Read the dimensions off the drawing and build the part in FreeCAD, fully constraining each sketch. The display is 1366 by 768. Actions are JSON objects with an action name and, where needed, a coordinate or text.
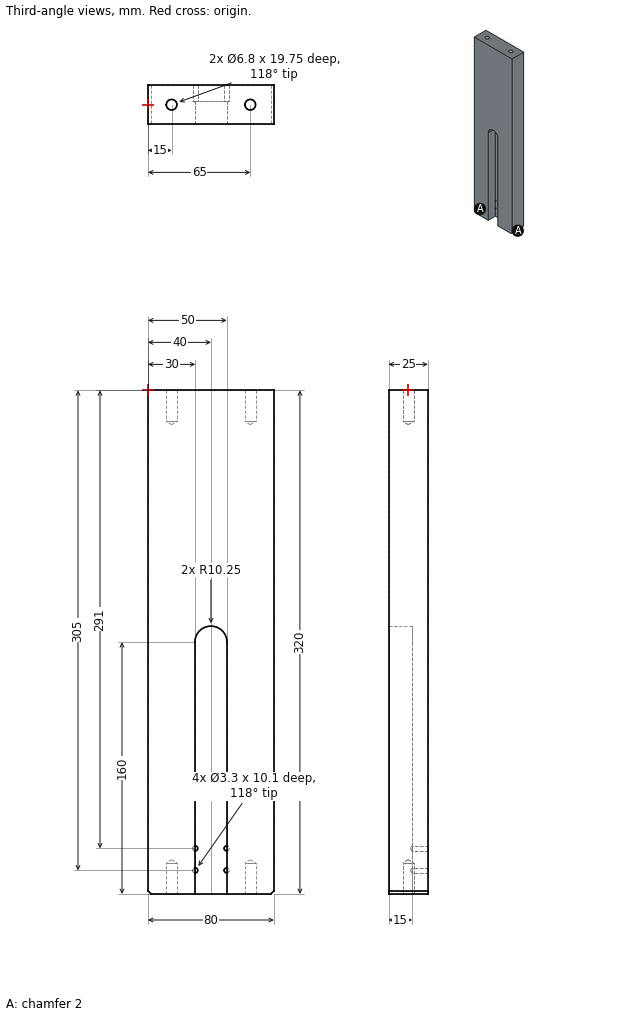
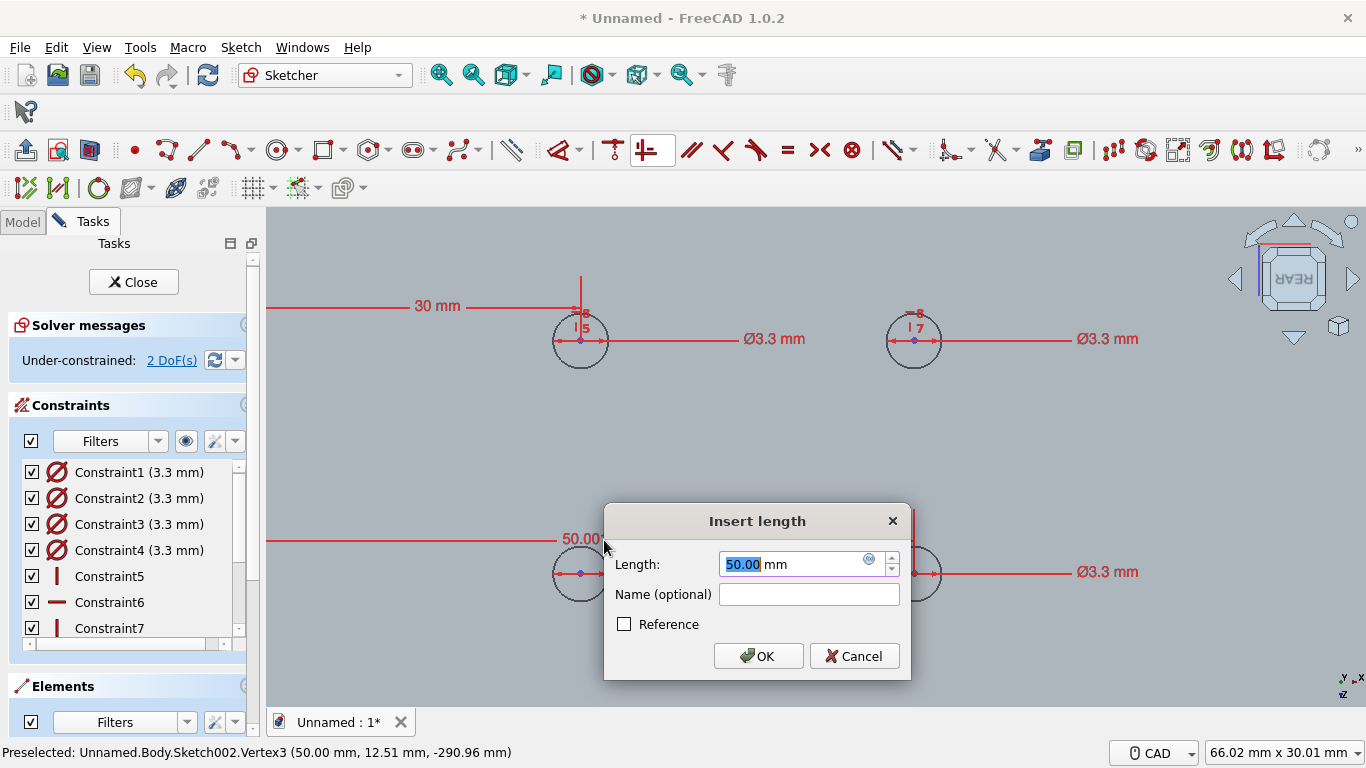
{"action": "type", "text": "50"}
{"action": "key", "text": "Return"}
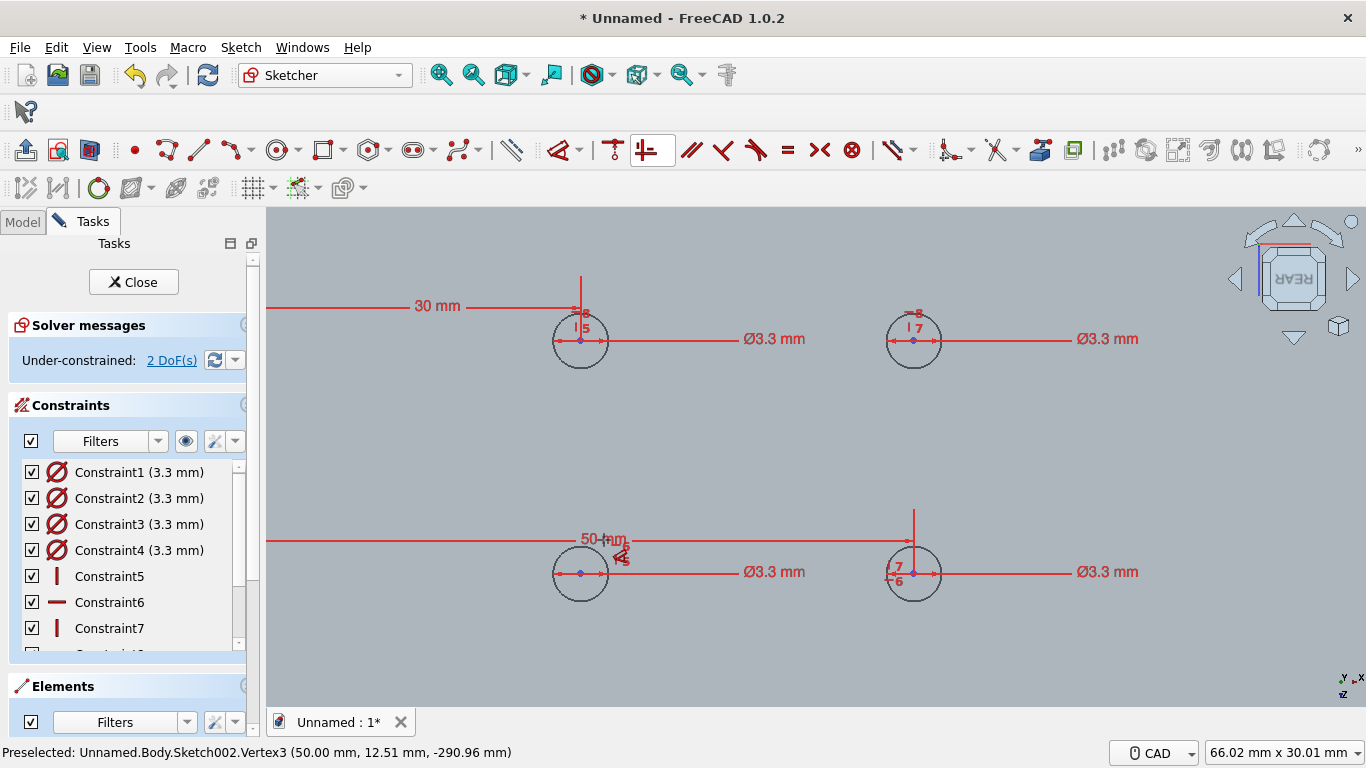
{"action": "left_click", "coordinate": [581, 341]}
{"action": "left_click", "coordinate": [615, 510]}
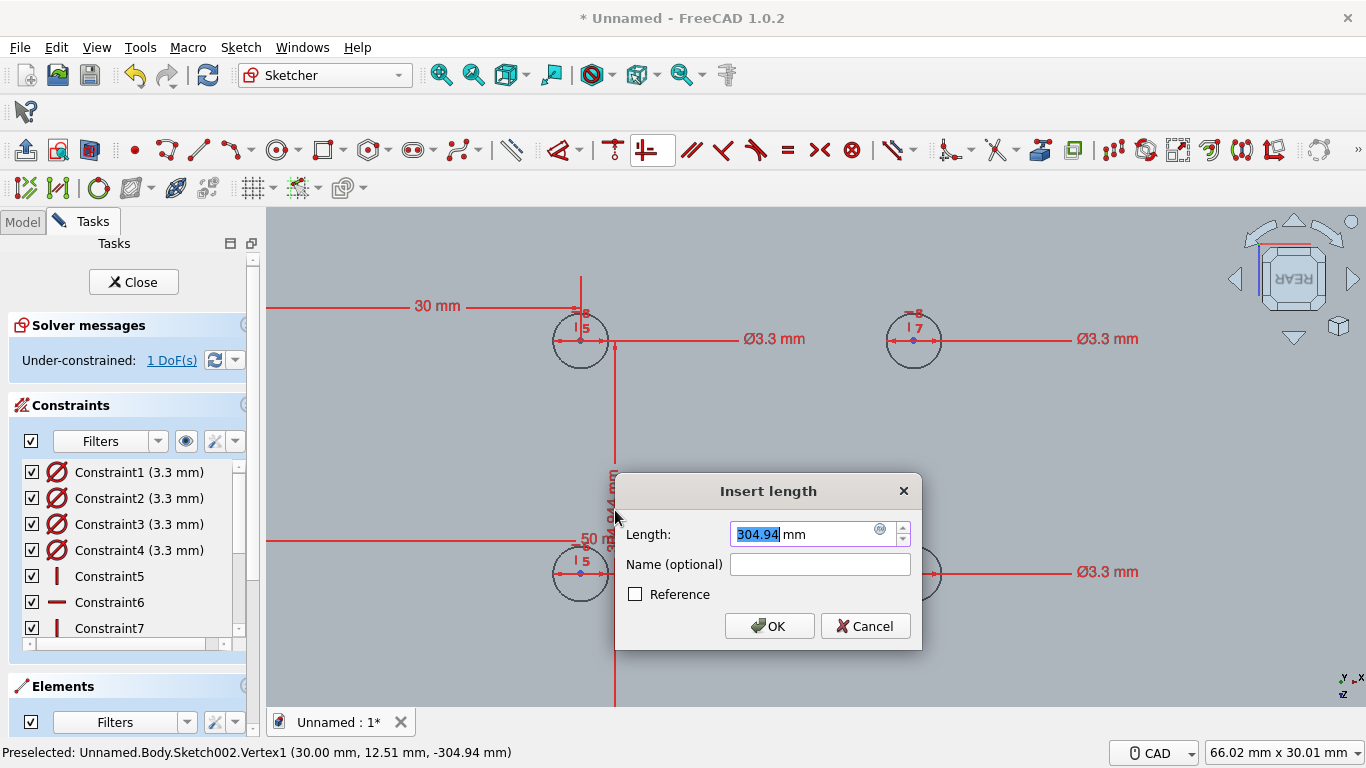
{"action": "type", "text": "305"}
{"action": "key", "text": "Return"}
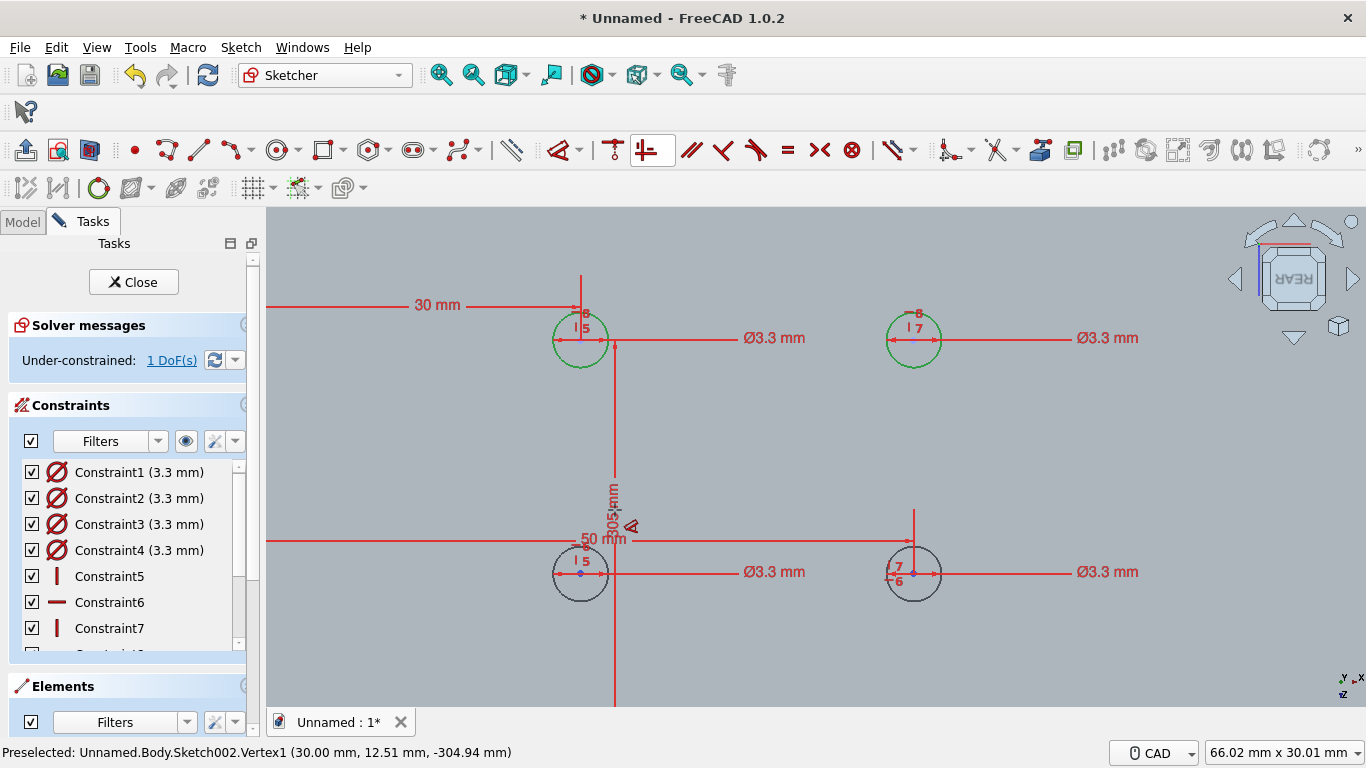
{"action": "left_click", "coordinate": [581, 574]}
{"action": "left_click", "coordinate": [615, 626]}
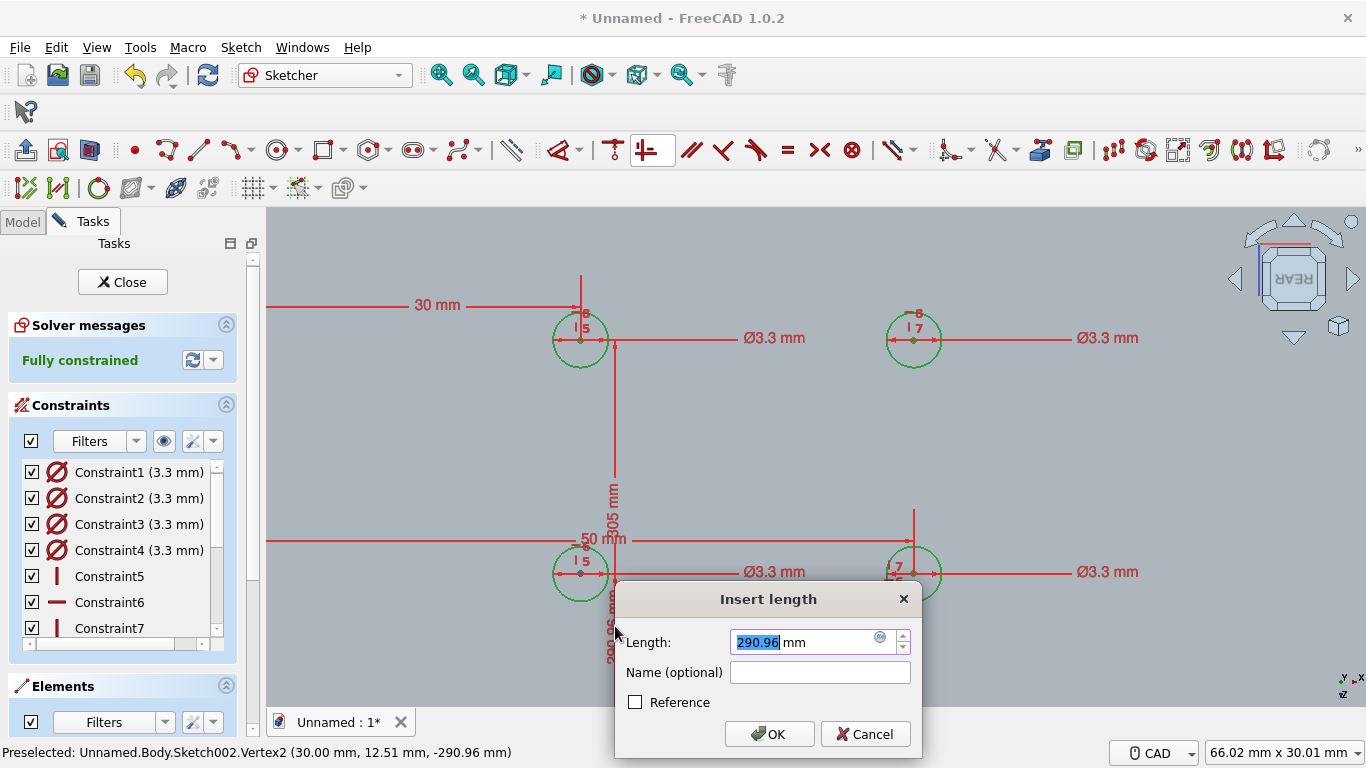
{"action": "type", "text": "291"}
{"action": "key", "text": "Return"}
{"action": "key", "text": "Escape"}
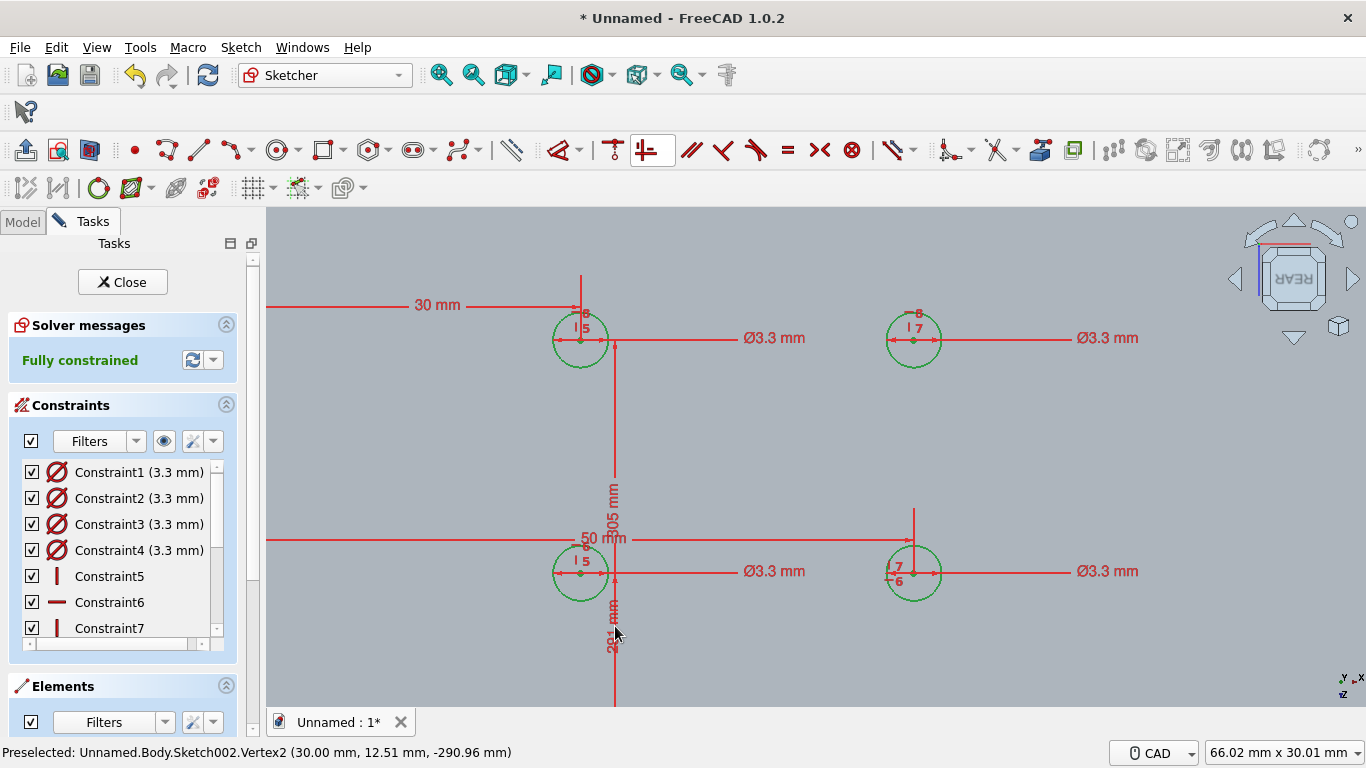
{"action": "left_click", "coordinate": [123, 282]}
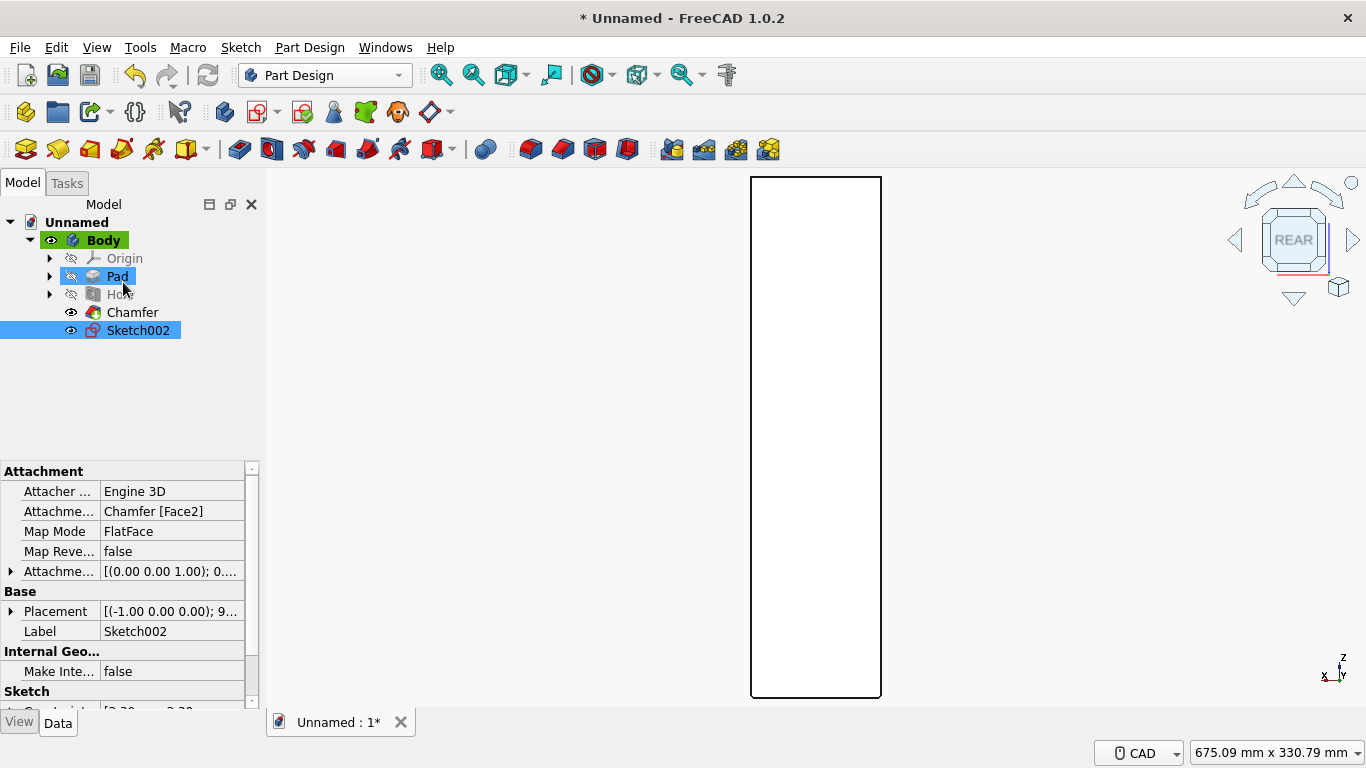
{"action": "left_click", "coordinate": [272, 150]}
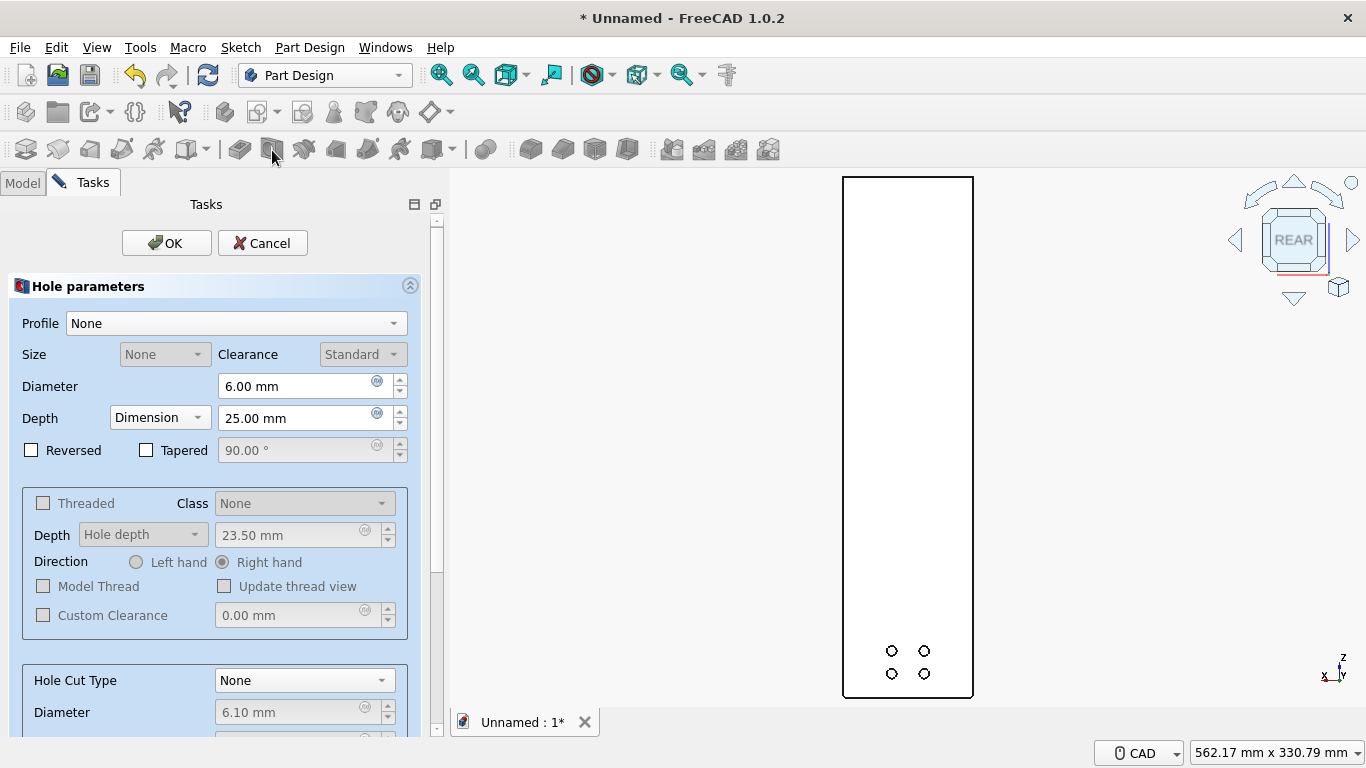
{"action": "triple_click", "coordinate": [305, 386]}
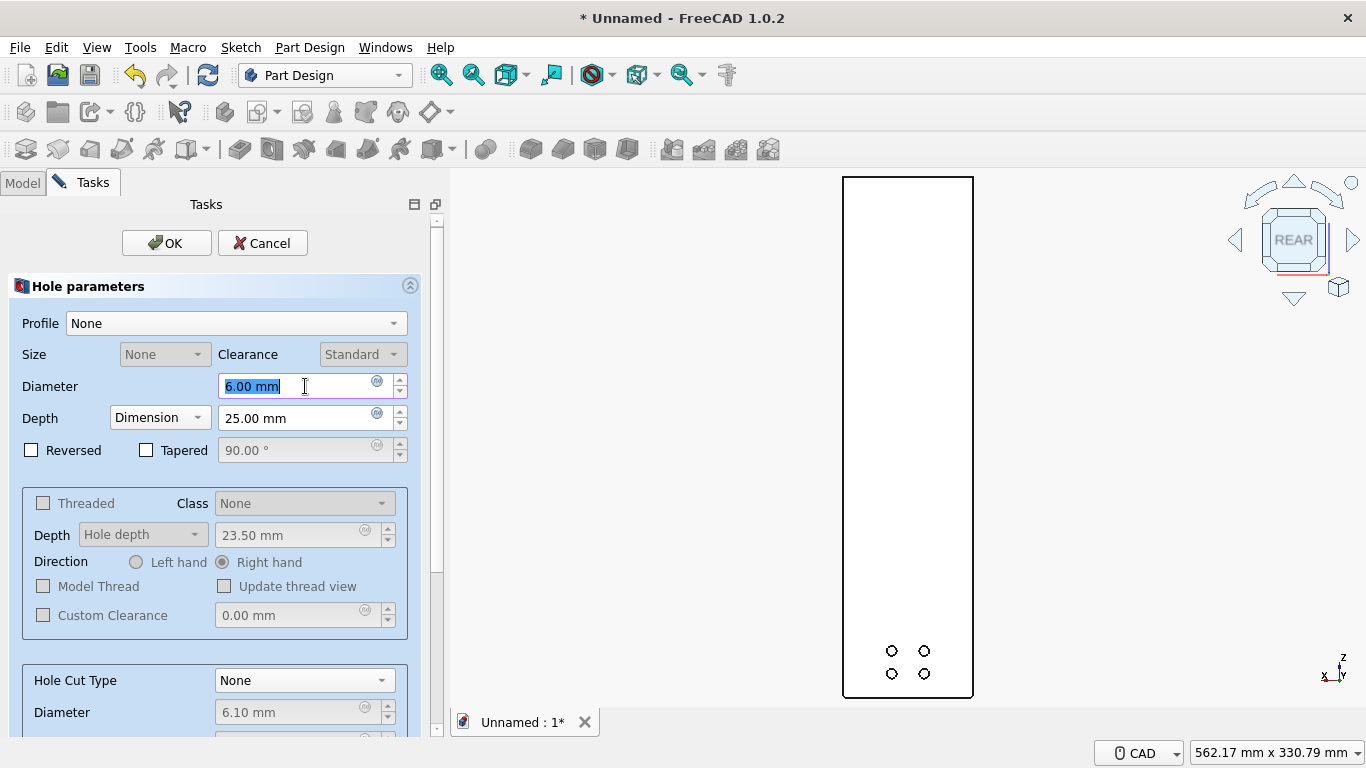
{"action": "type", "text": "3.3"}
{"action": "key", "text": "Tab"}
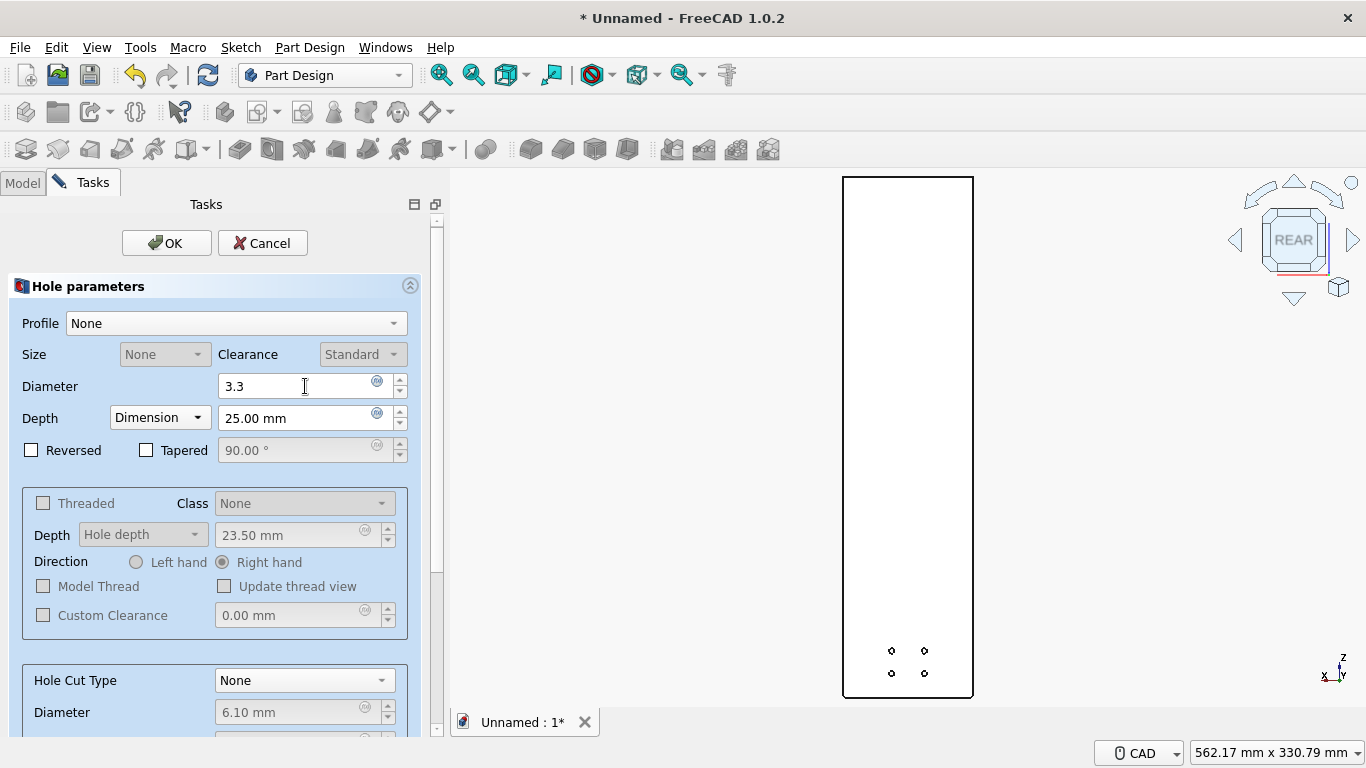
{"action": "triple_click", "coordinate": [305, 418]}